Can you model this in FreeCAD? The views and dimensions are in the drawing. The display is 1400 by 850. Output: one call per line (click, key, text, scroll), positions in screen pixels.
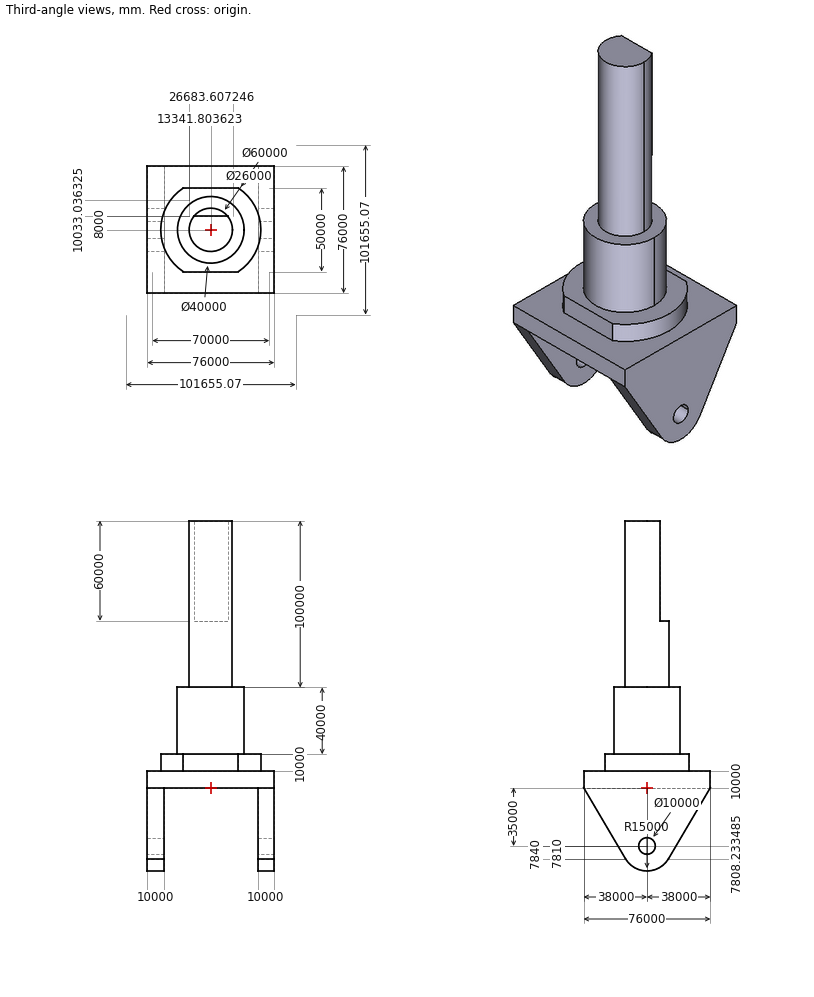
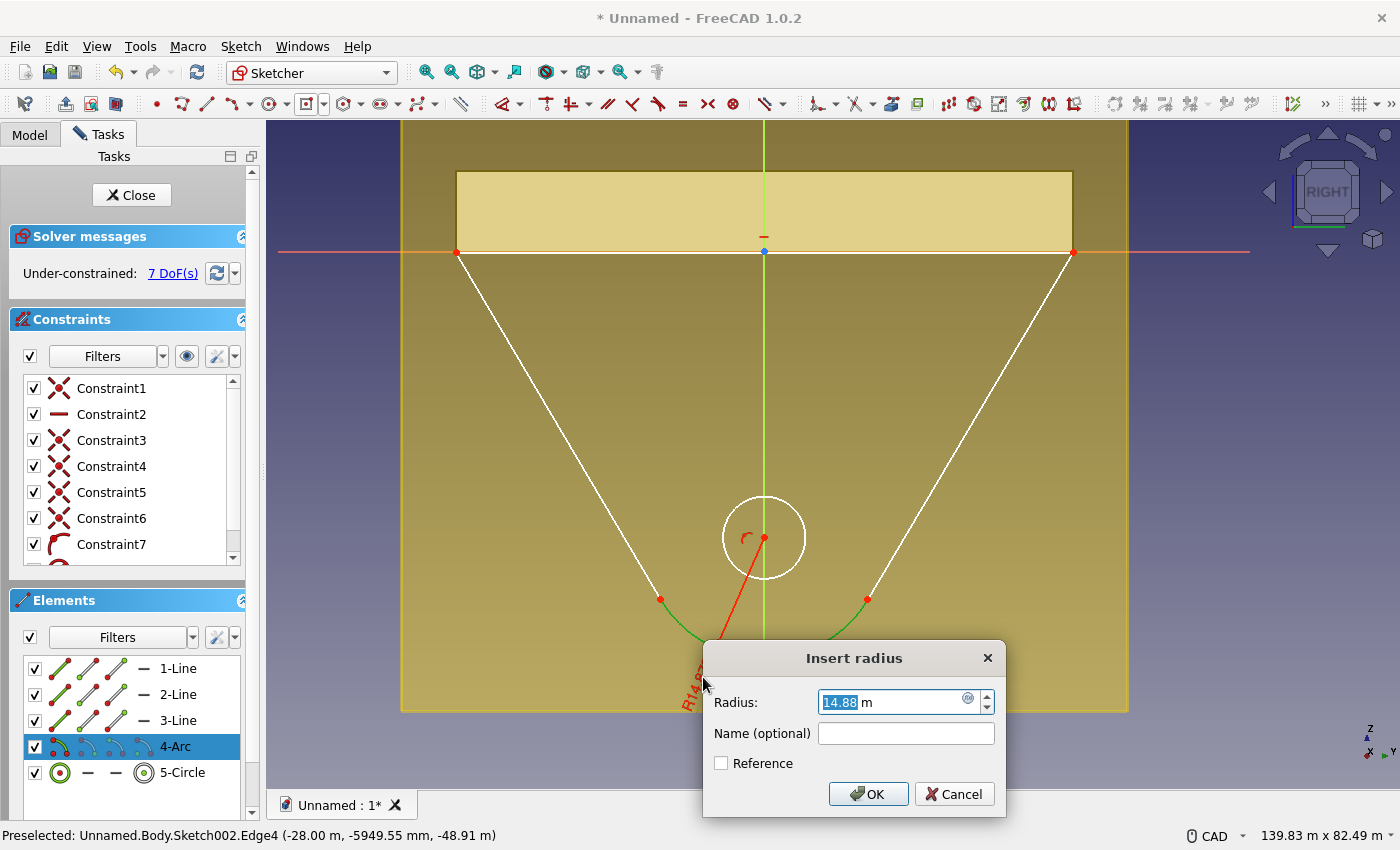
key(ctrl+a)
text(15000 mm)
key(Return)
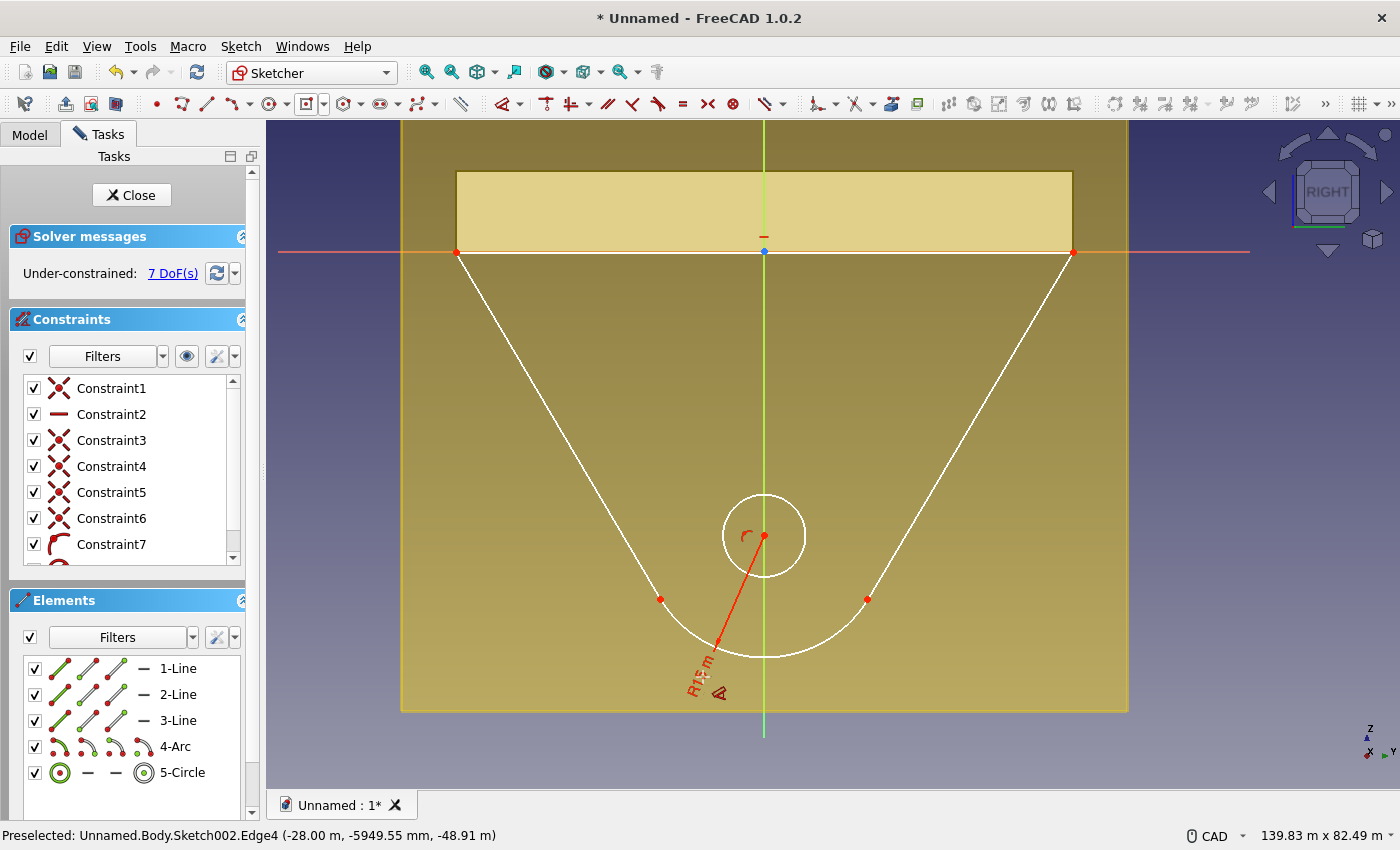
click(793, 507)
click(816, 484)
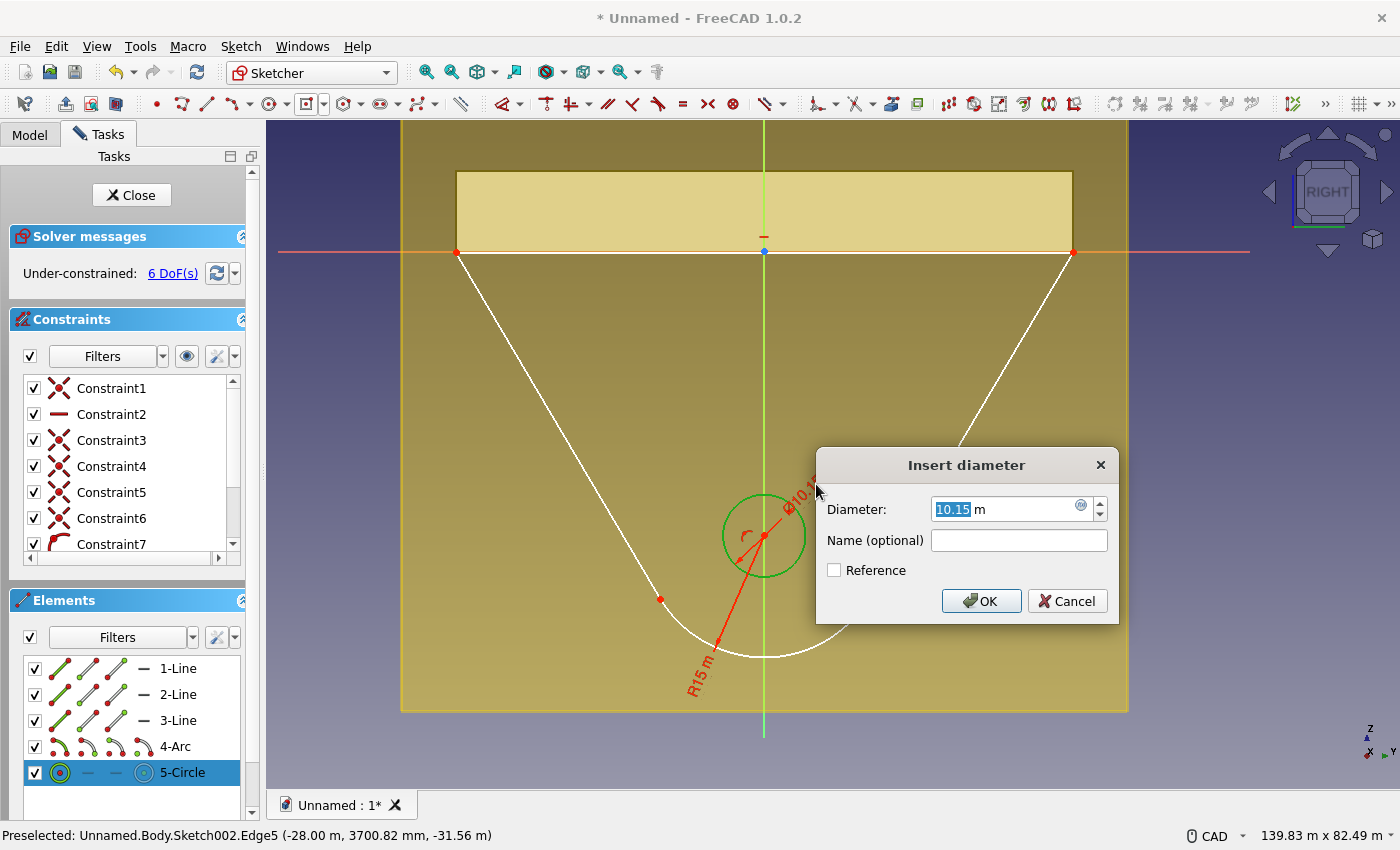
key(ctrl+a)
text(10000 mm)
key(Return)
key(Escape)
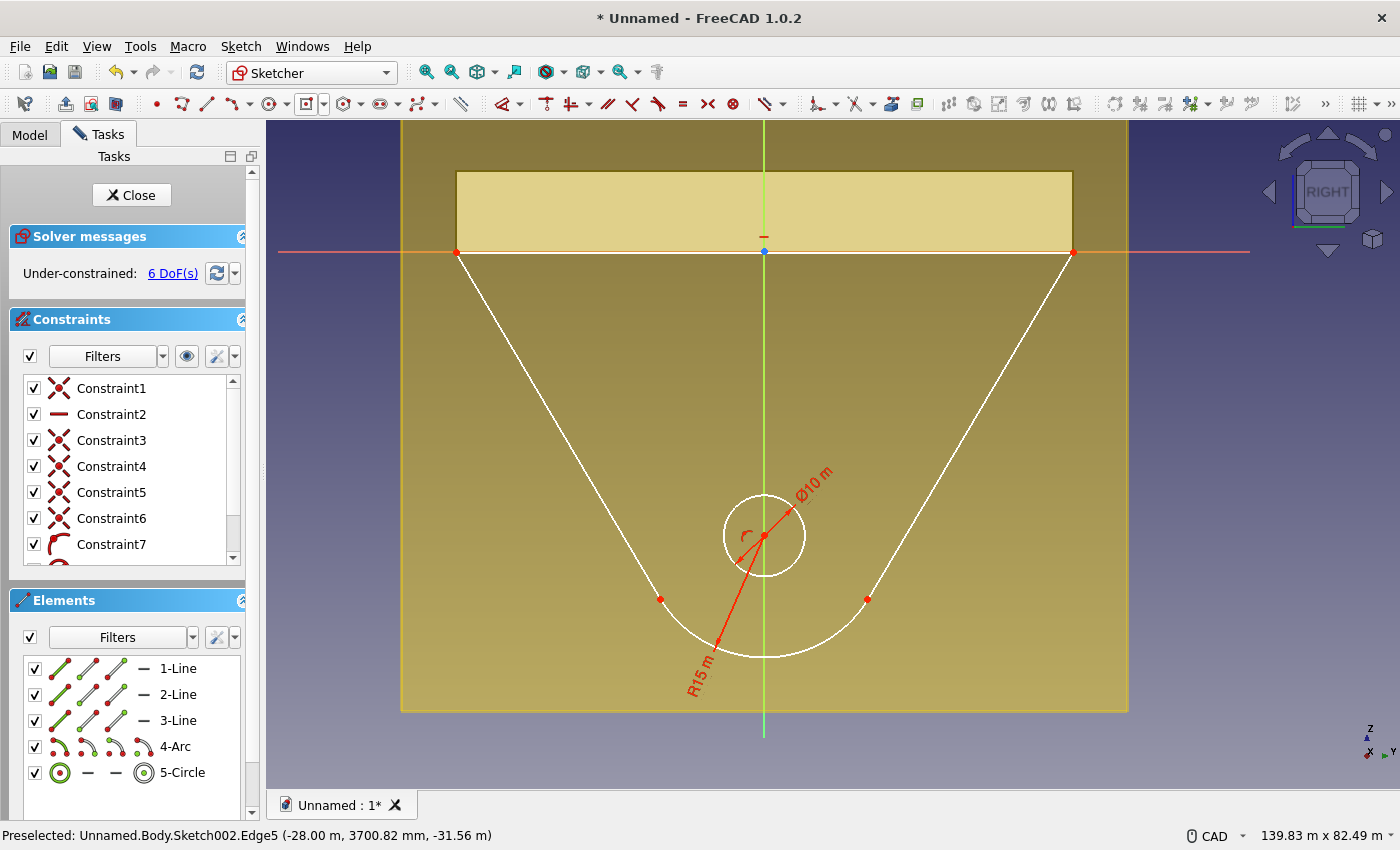
click(456, 253)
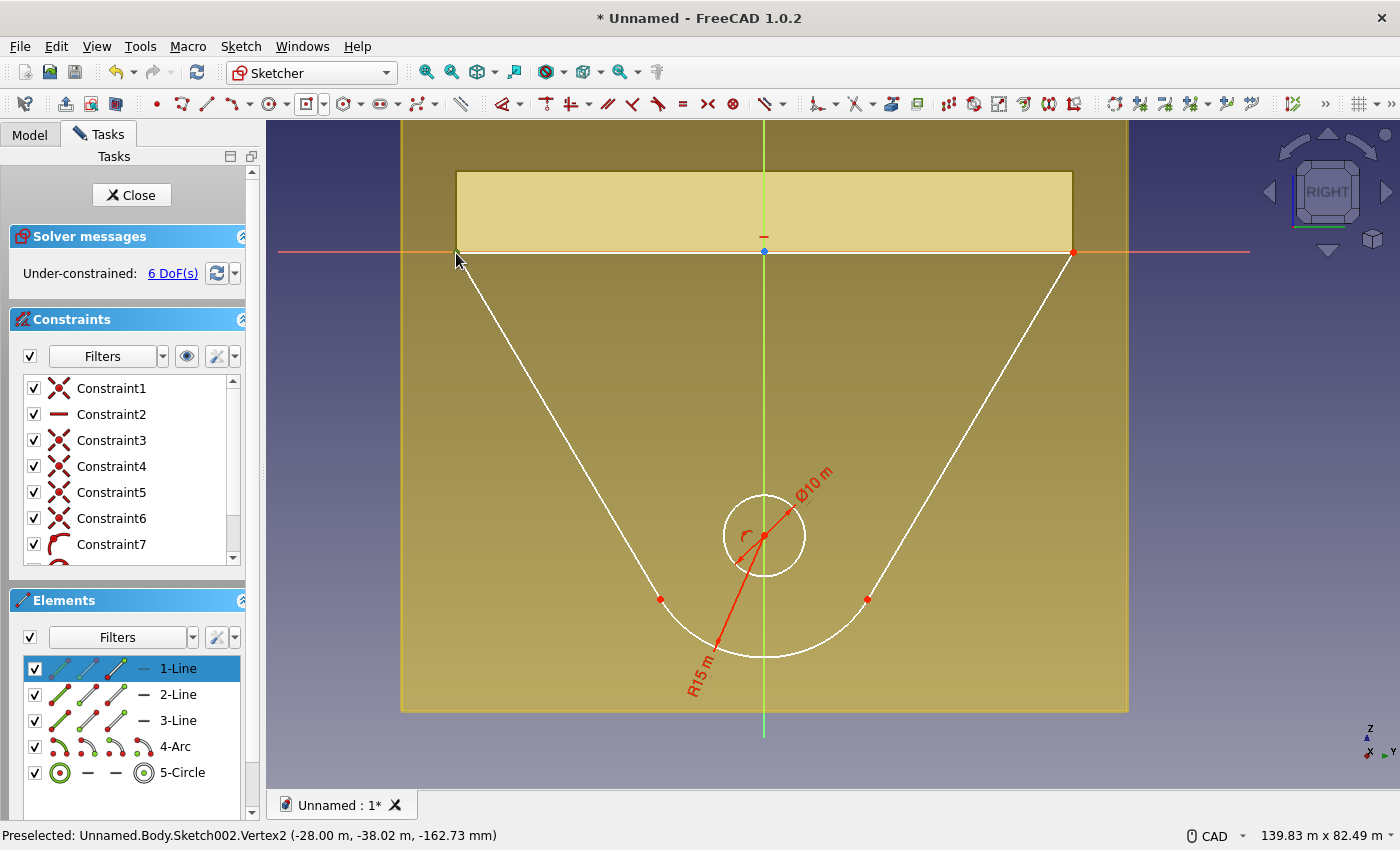
click(361, 252)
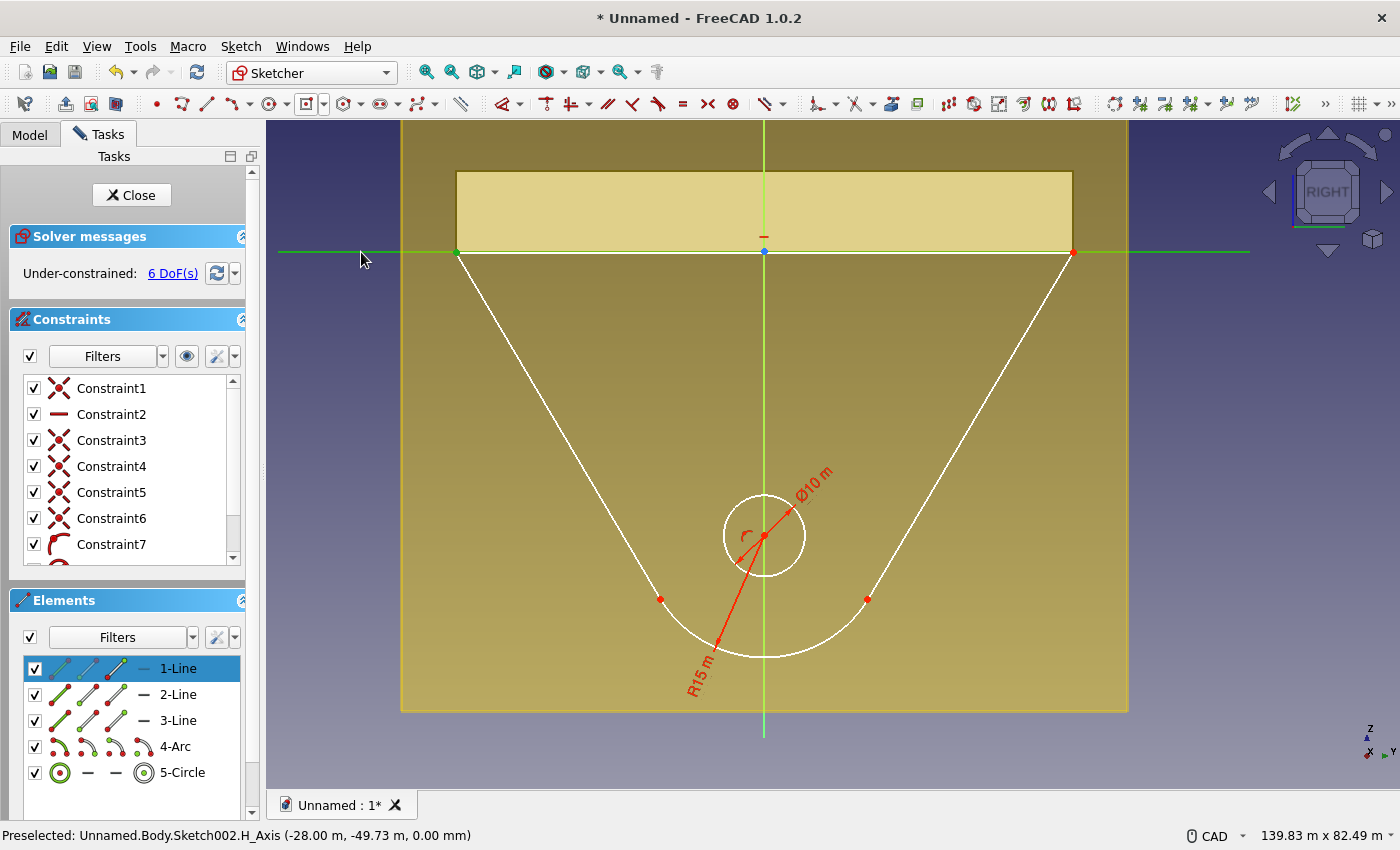
click(546, 104)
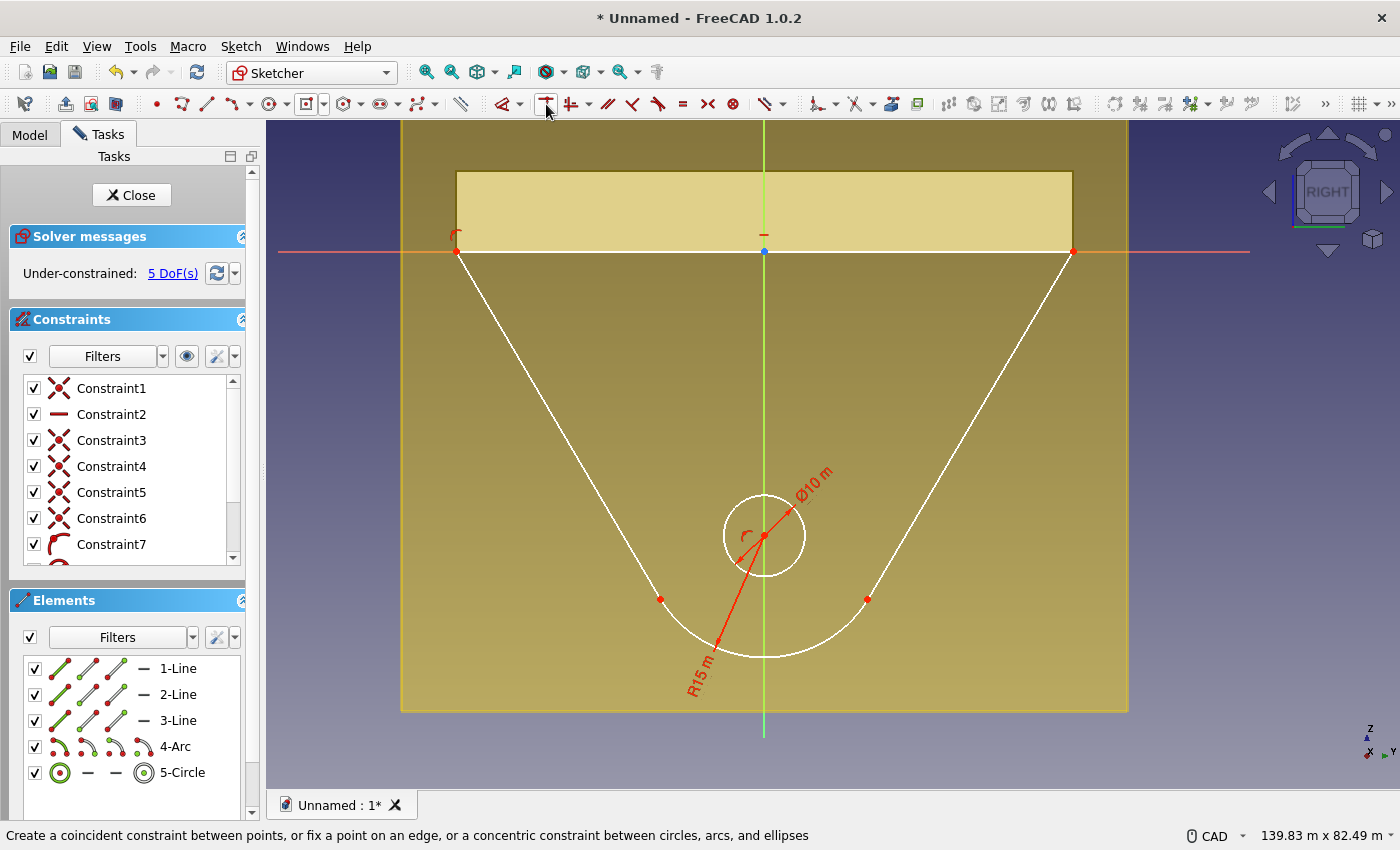
click(502, 104)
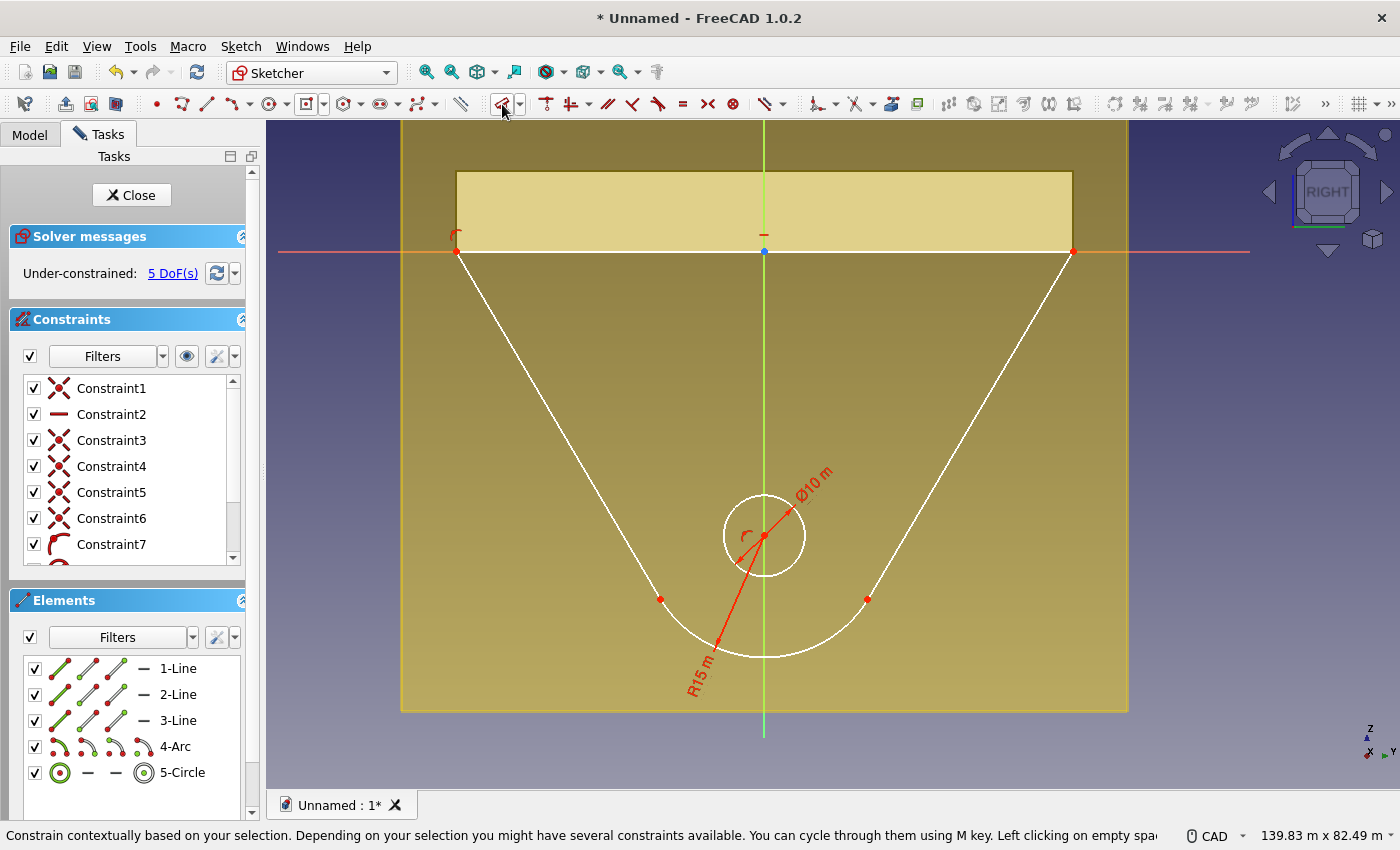
click(641, 252)
click(623, 218)